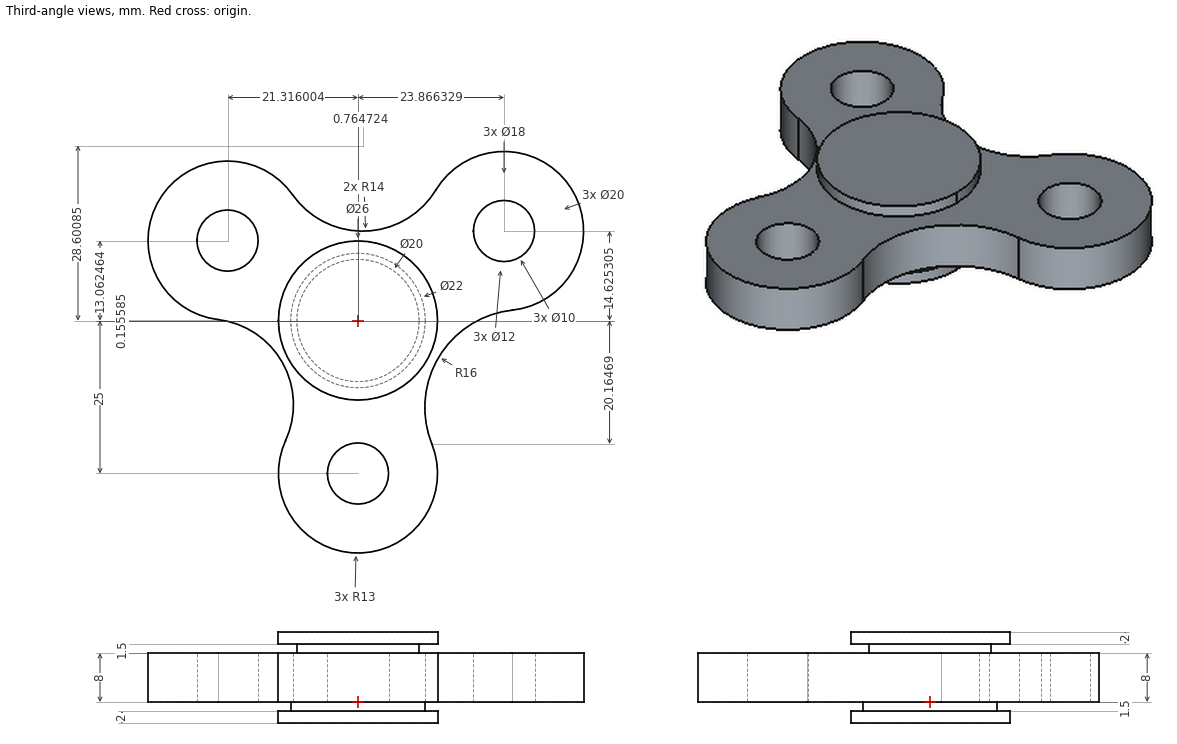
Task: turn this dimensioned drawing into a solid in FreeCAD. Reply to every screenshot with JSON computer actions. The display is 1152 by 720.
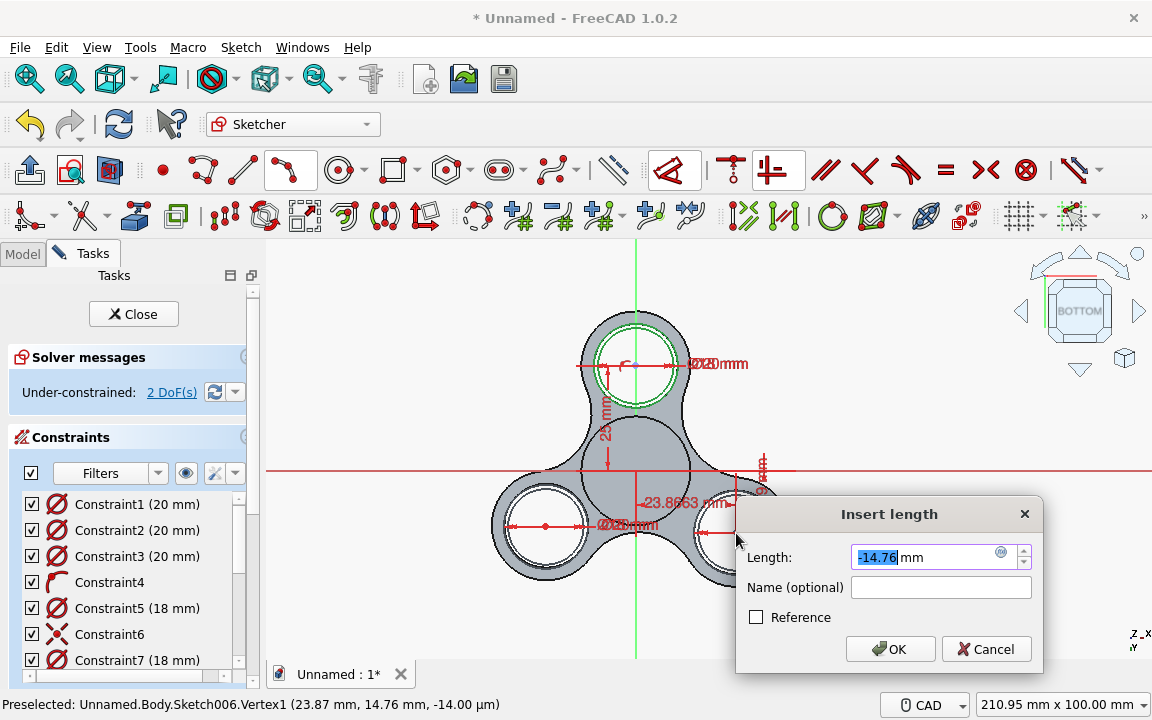
{"action": "type", "text": "-14.625305"}
{"action": "key", "text": "Return"}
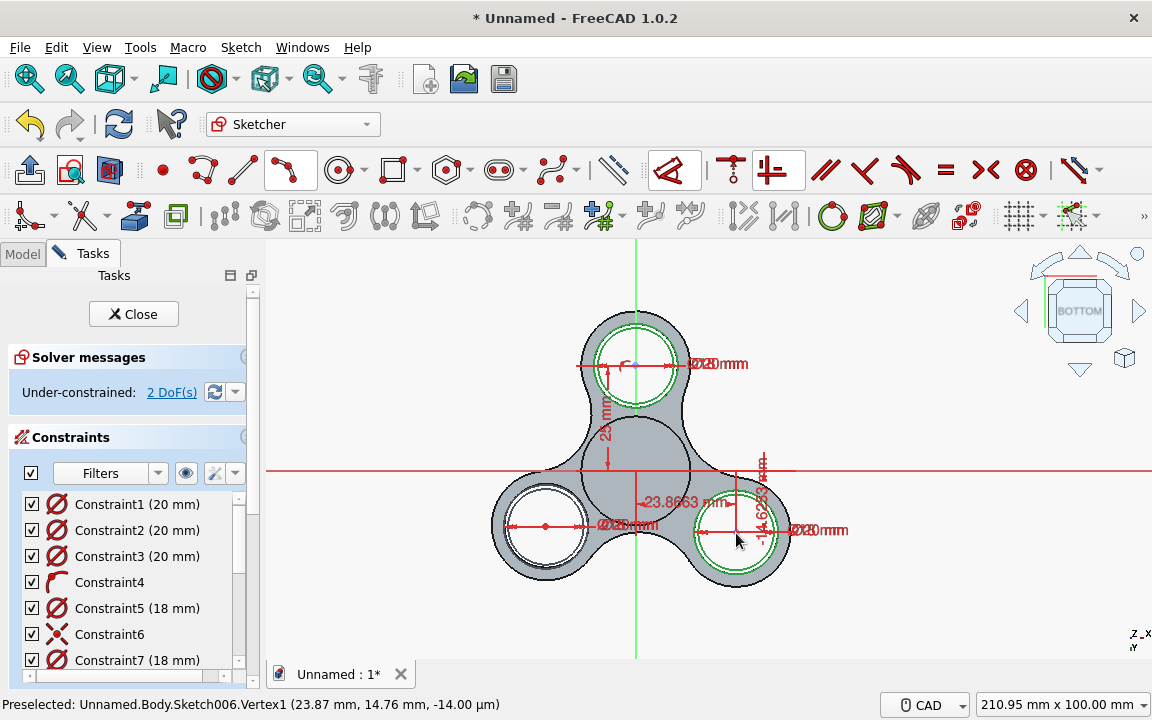
{"action": "left_click", "coordinate": [546, 527]}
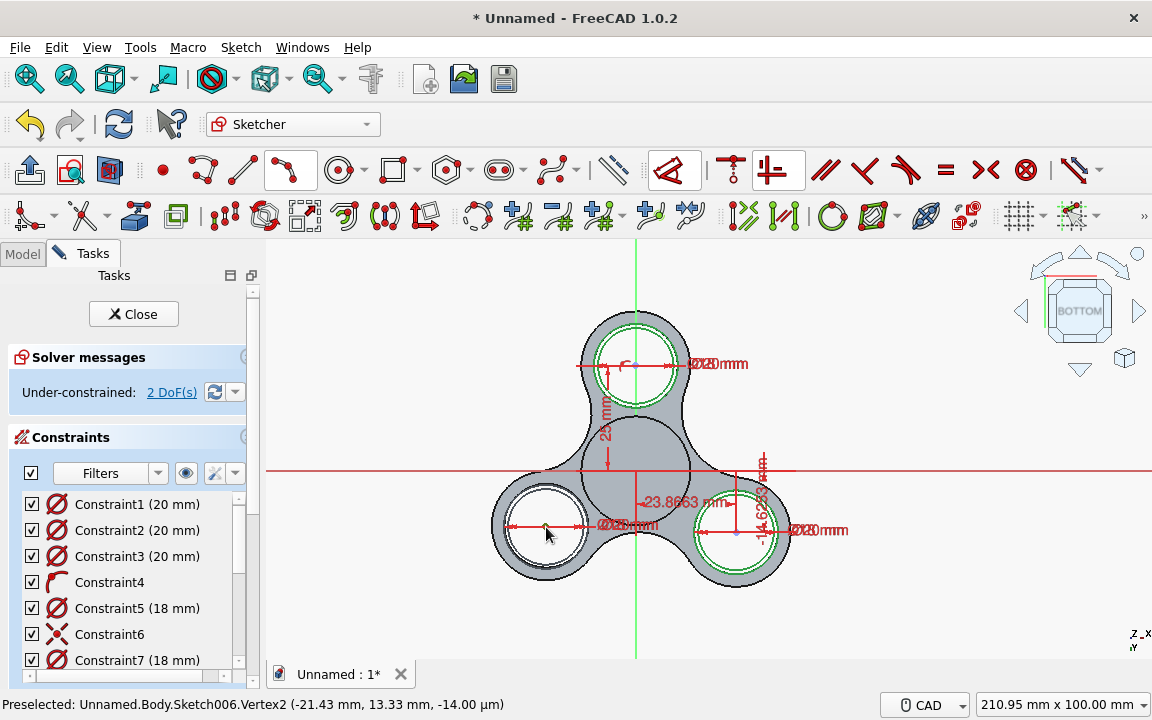
{"action": "key", "text": "l"}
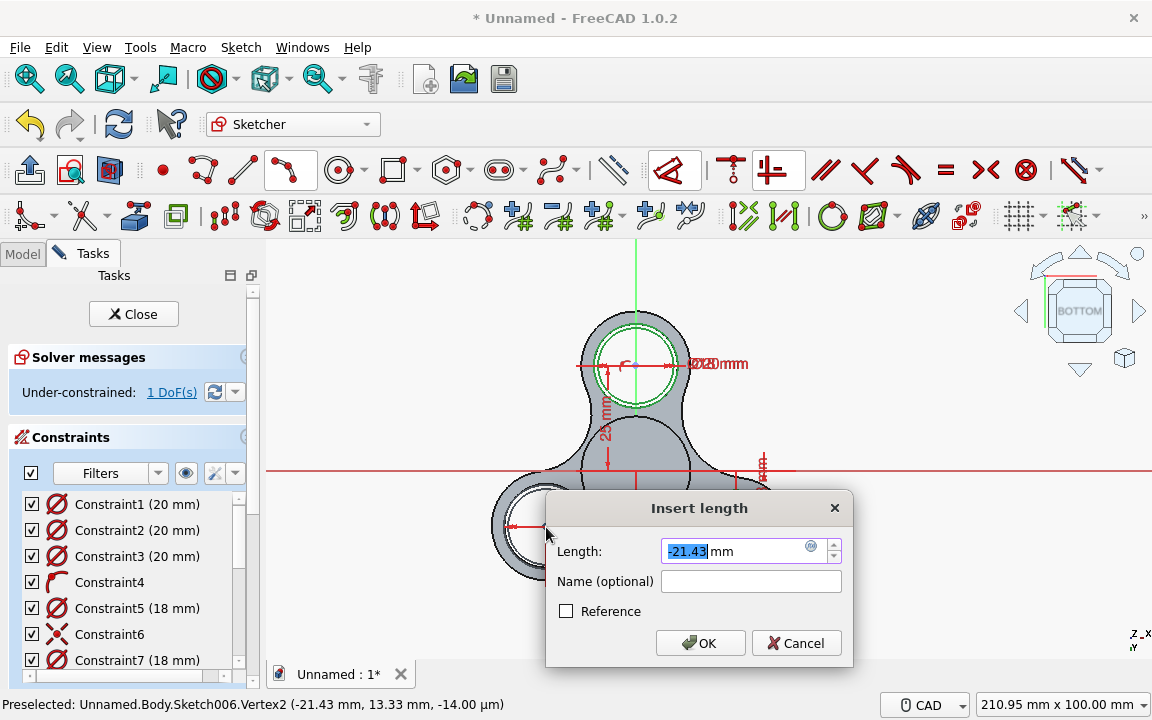
{"action": "type", "text": "-21.316004"}
{"action": "key", "text": "Return"}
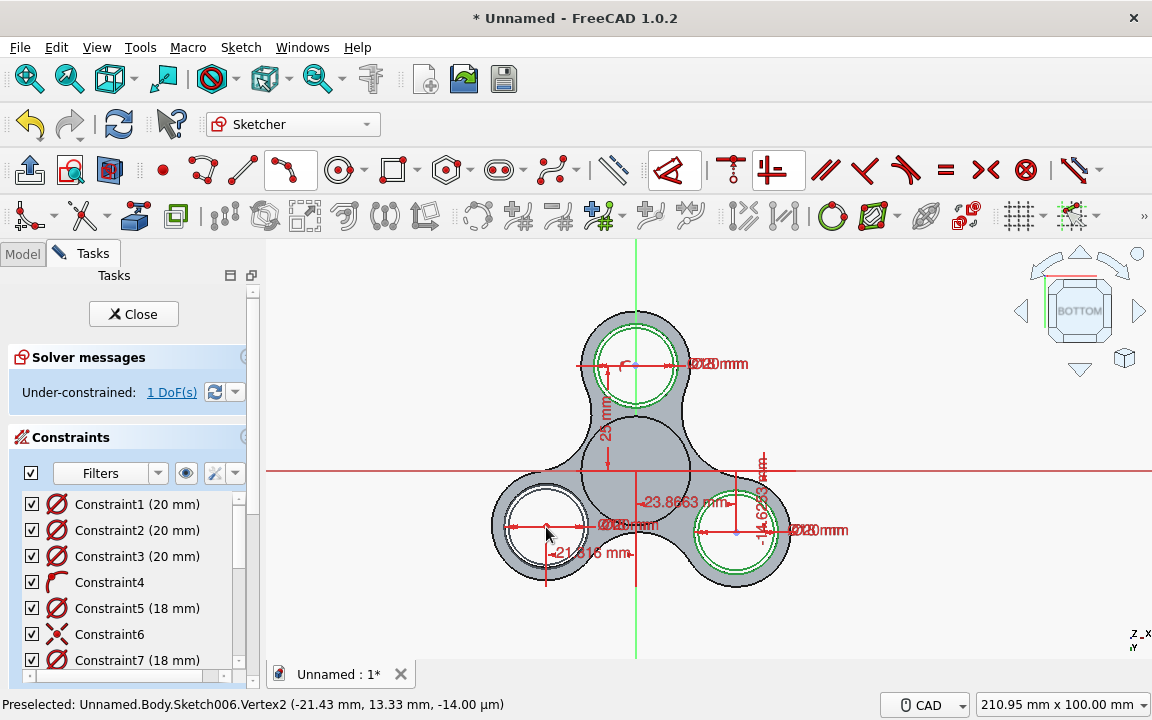
{"action": "left_click", "coordinate": [546, 527]}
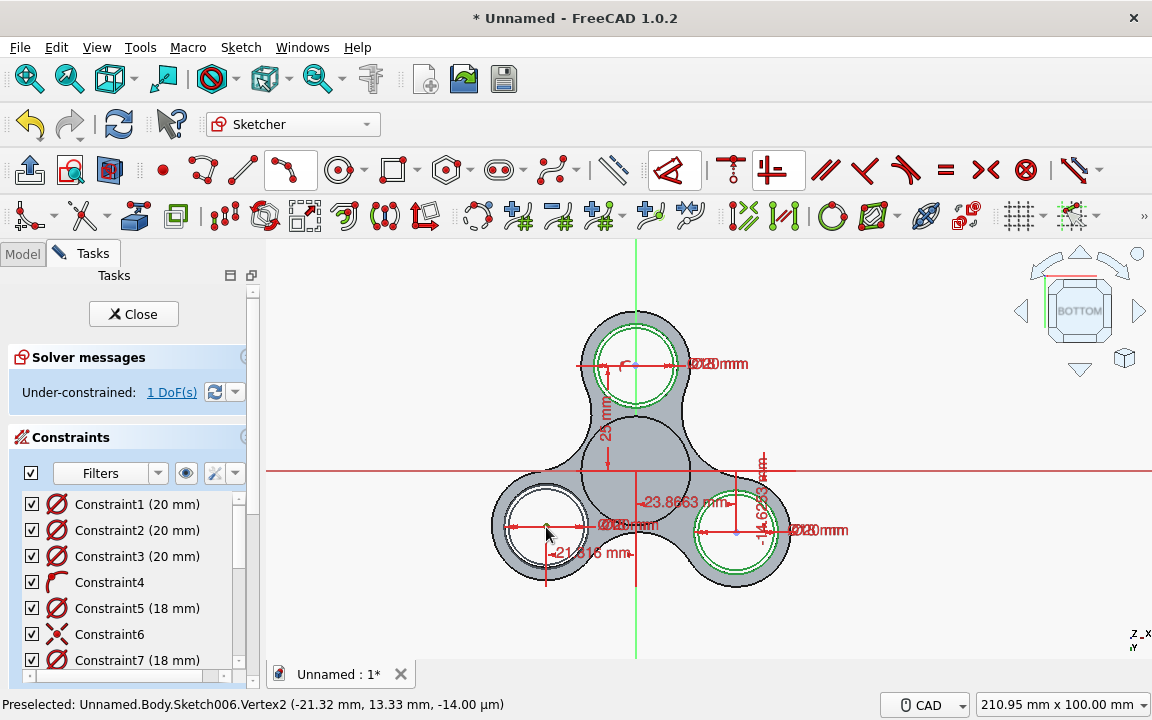
{"action": "key", "text": "i"}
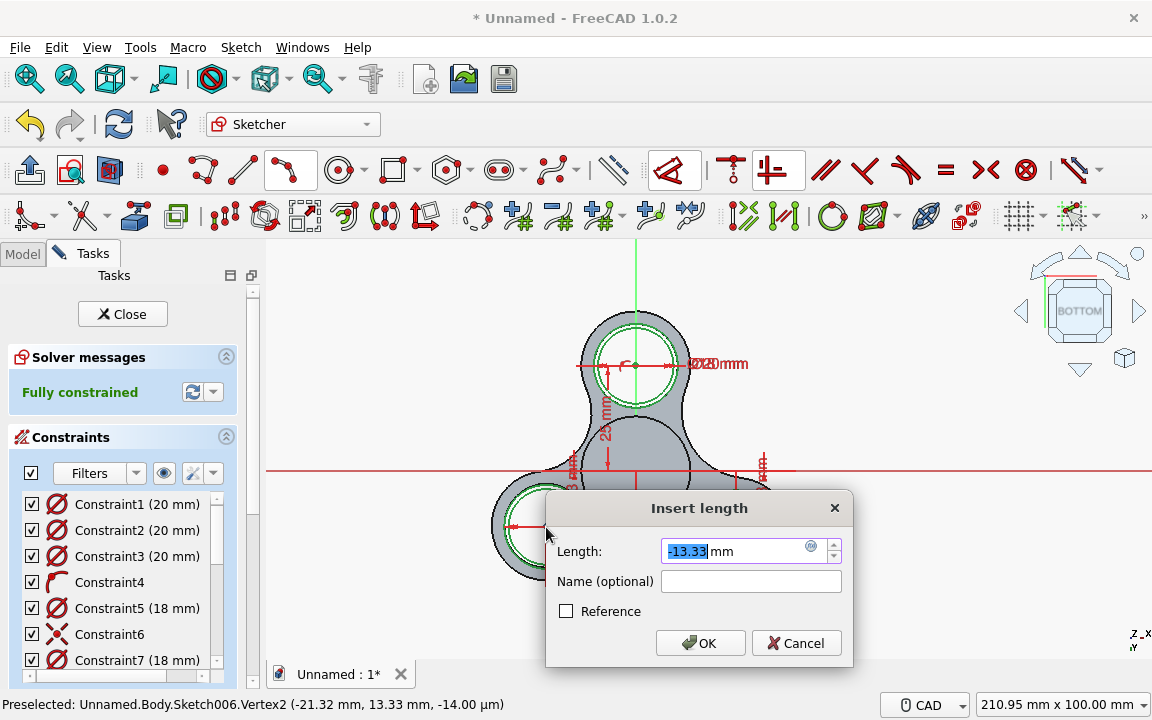
{"action": "type", "text": "-13.062464"}
{"action": "key", "text": "Return"}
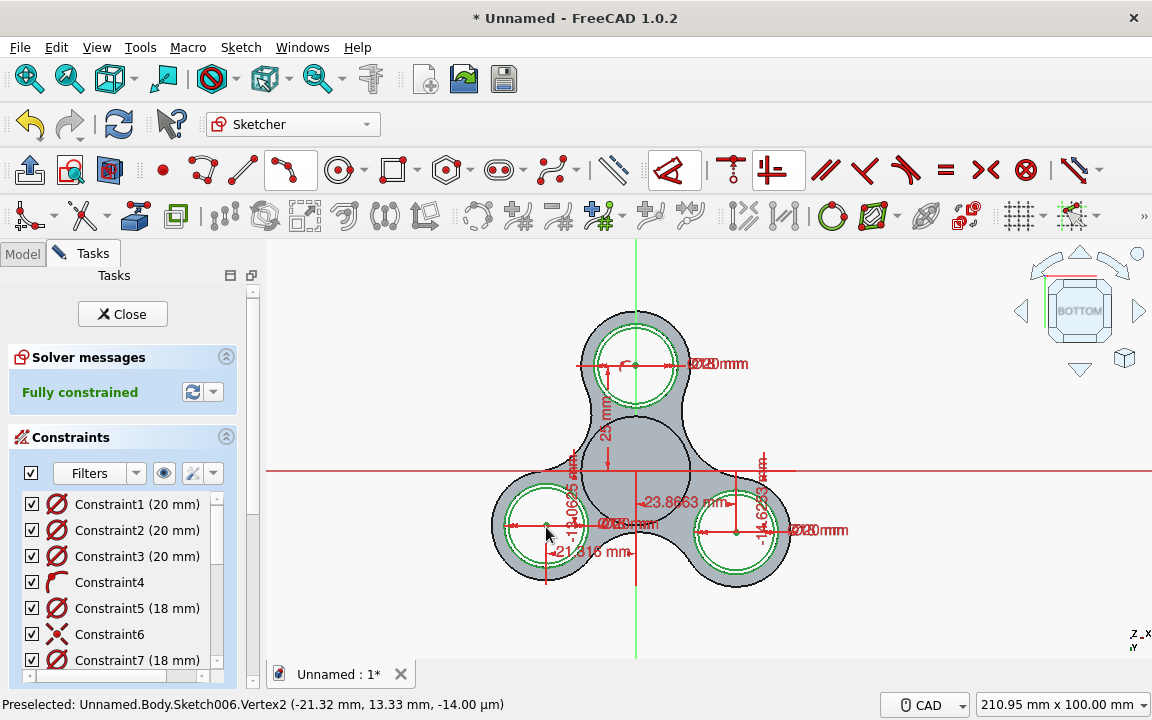
{"action": "left_click", "coordinate": [123, 314]}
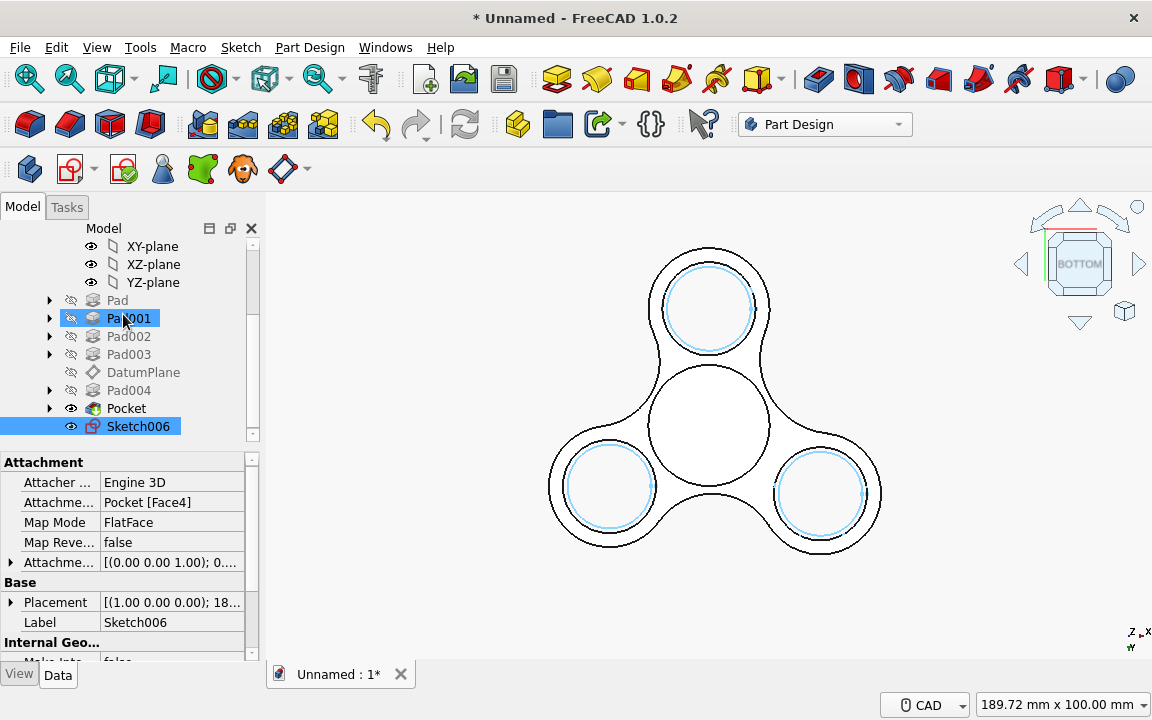
{"action": "left_click", "coordinate": [558, 80]}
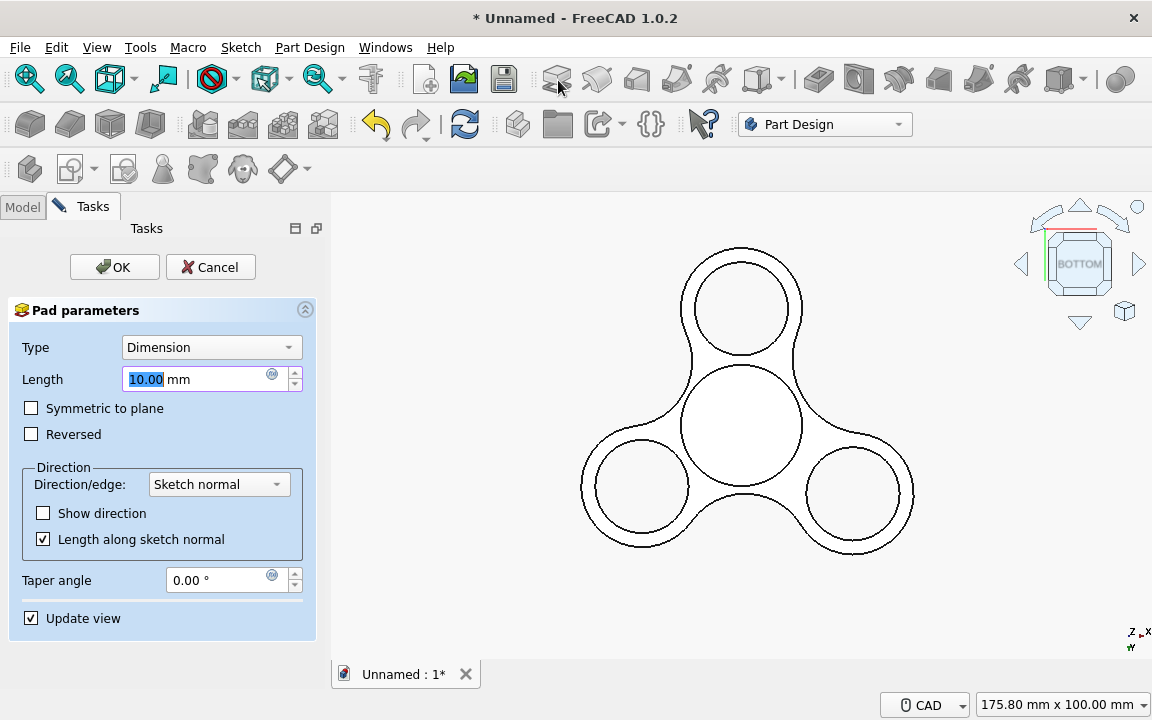
{"action": "type", "text": "8"}
{"action": "key", "text": "Tab"}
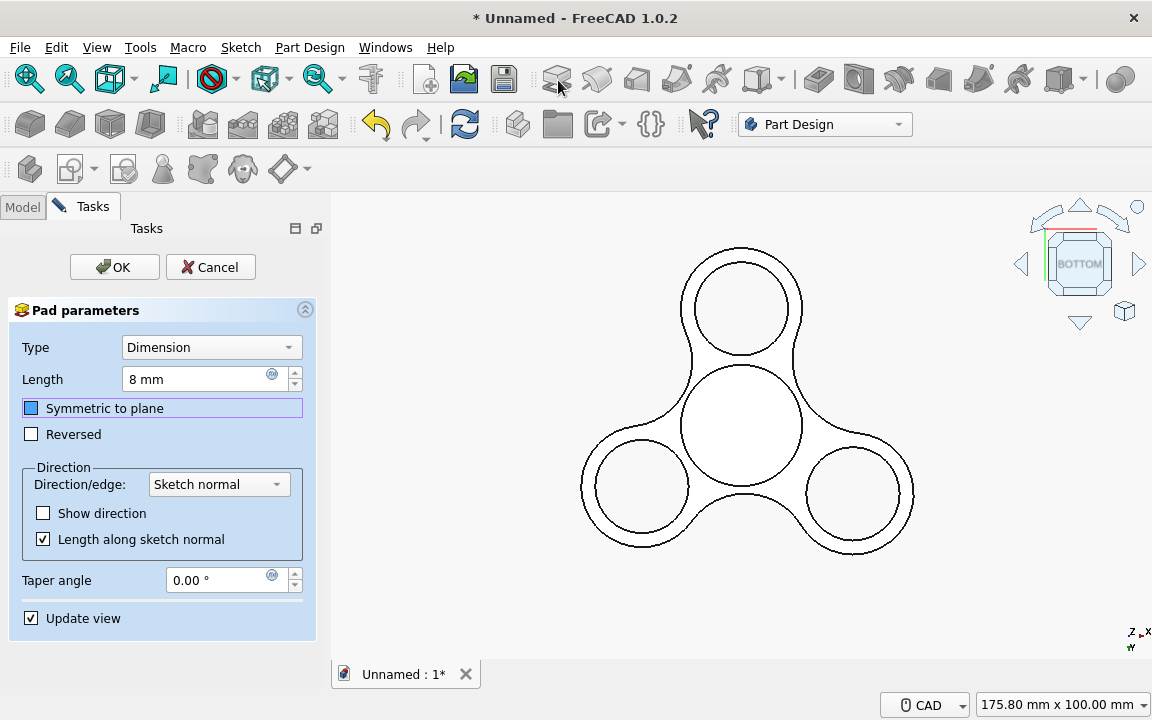
{"action": "left_click", "coordinate": [30, 434]}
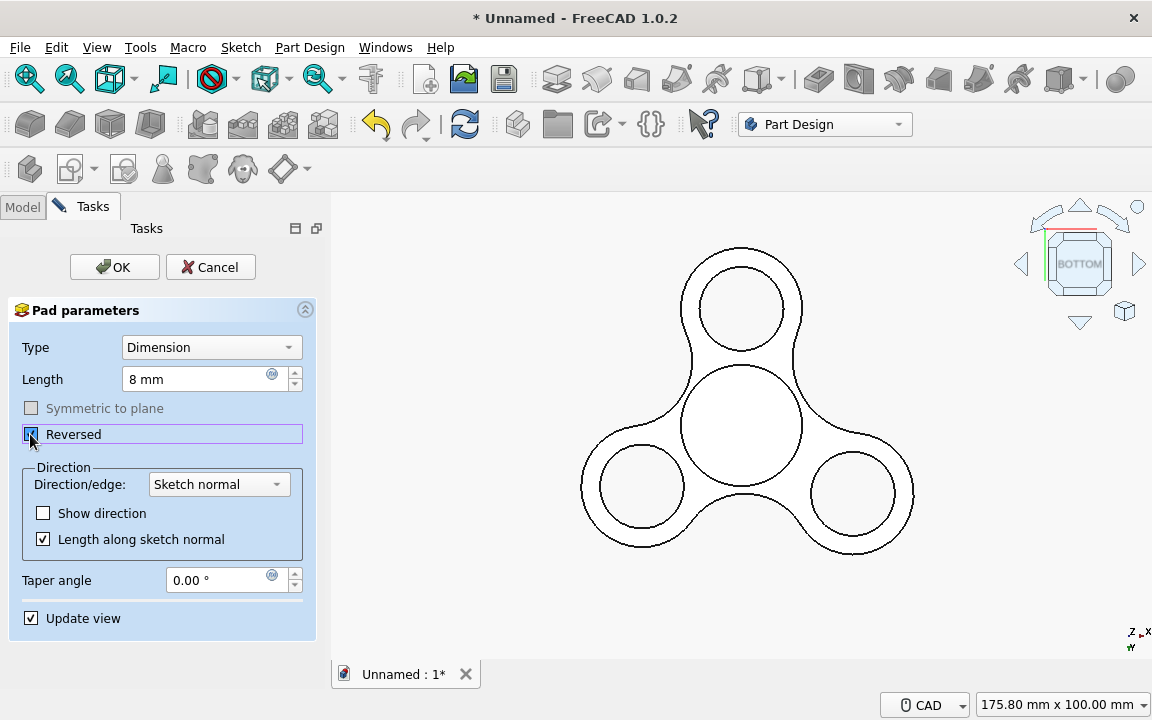
{"action": "left_click", "coordinate": [115, 267]}